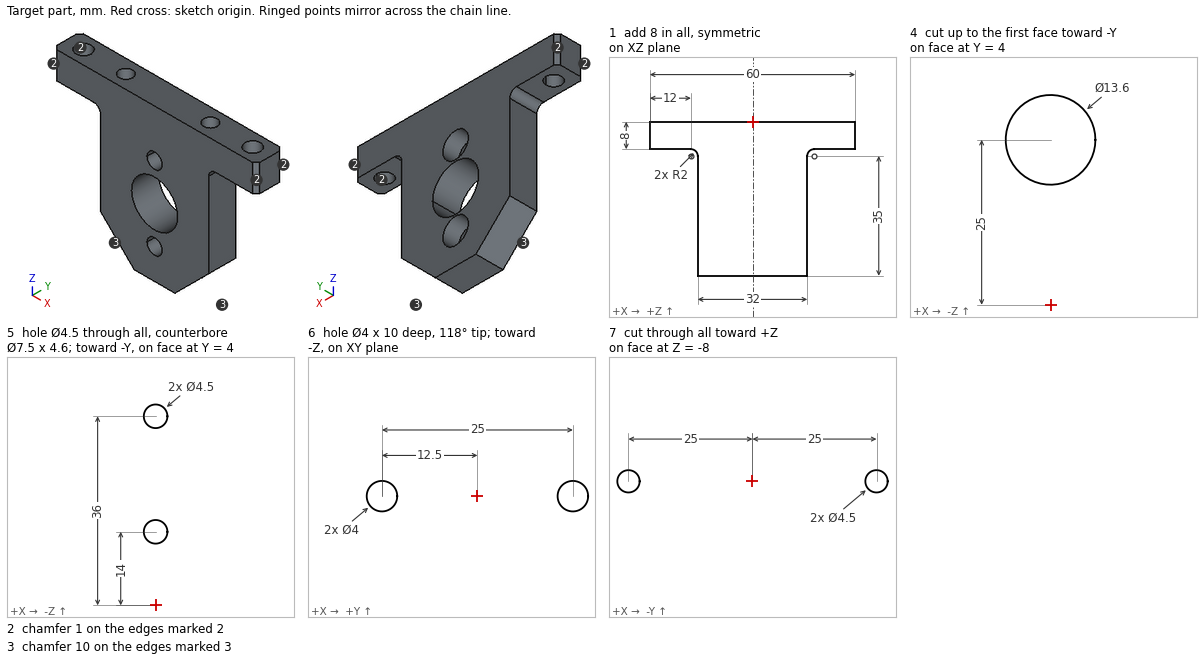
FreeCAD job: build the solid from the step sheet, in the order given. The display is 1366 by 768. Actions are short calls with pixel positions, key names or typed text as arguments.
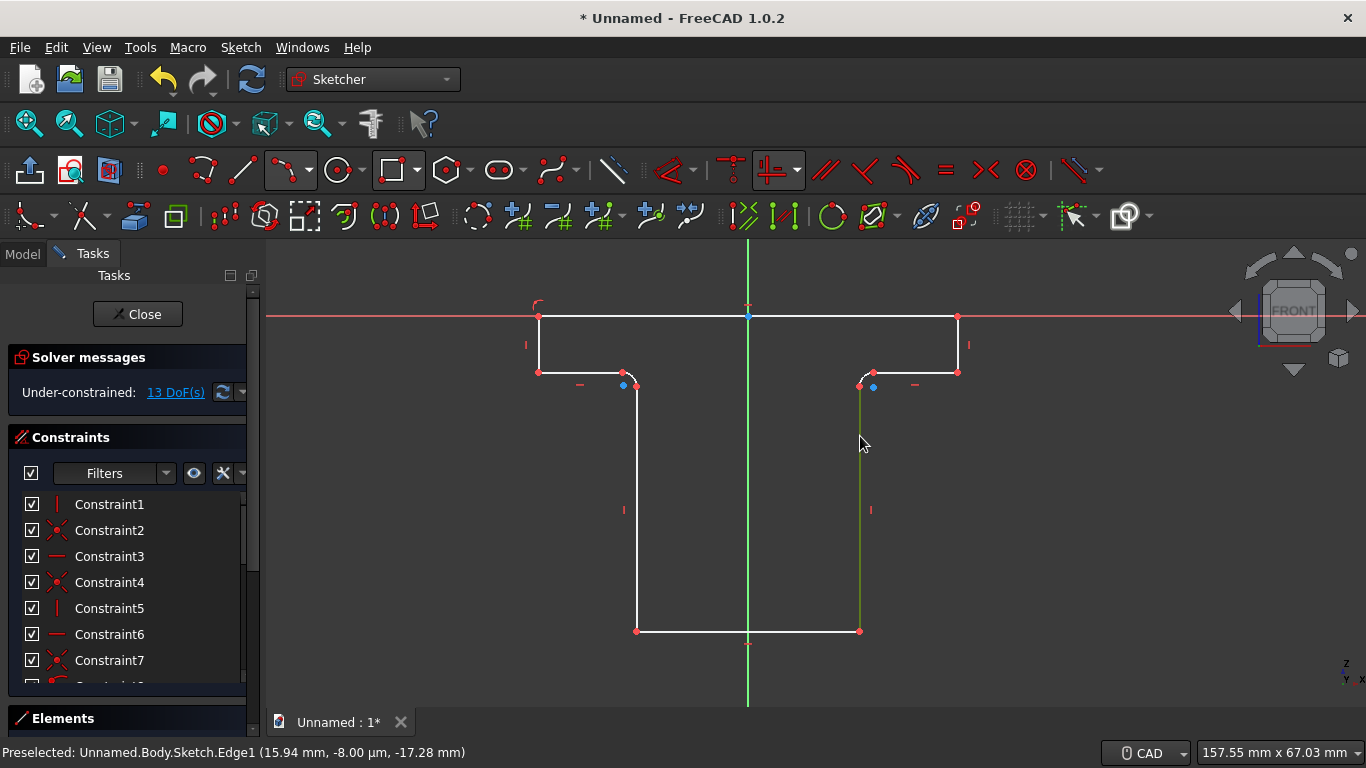
scroll(864, 377, up, 2)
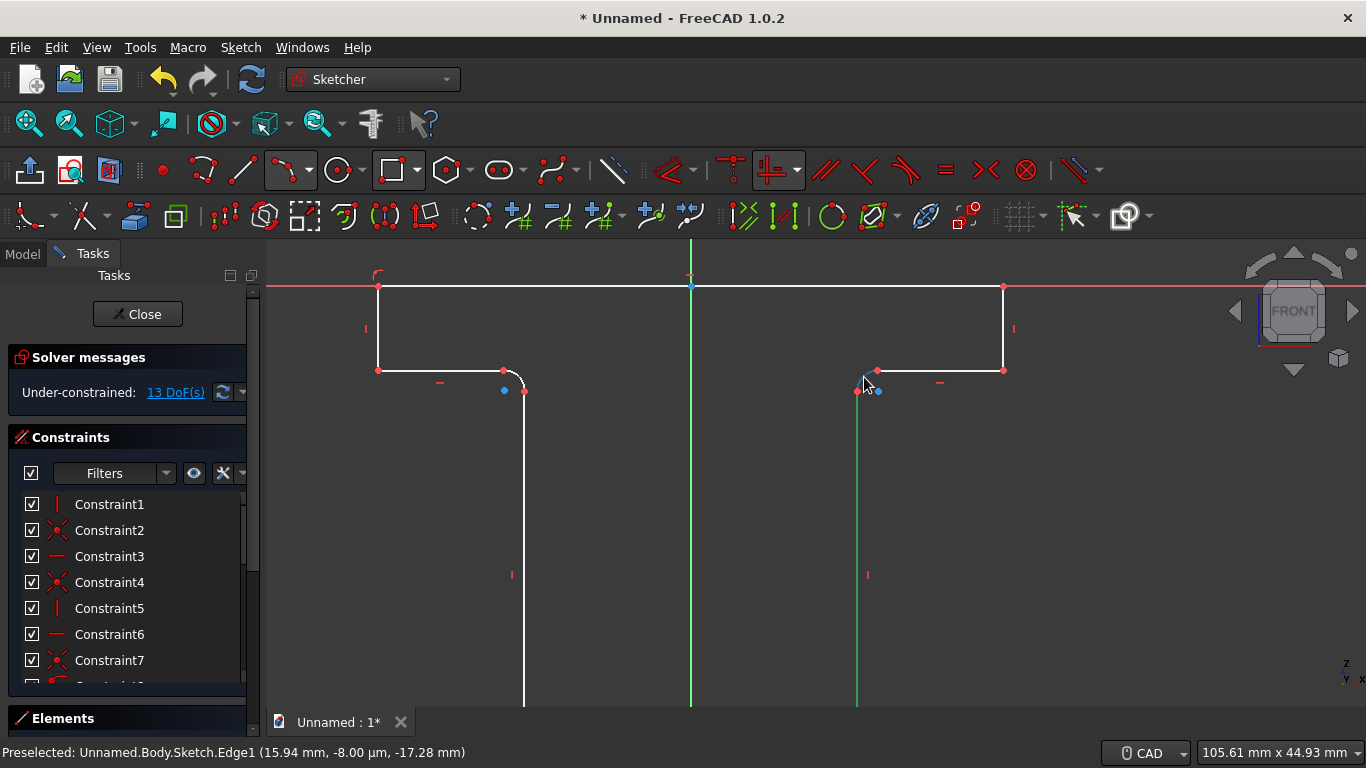
click(863, 377)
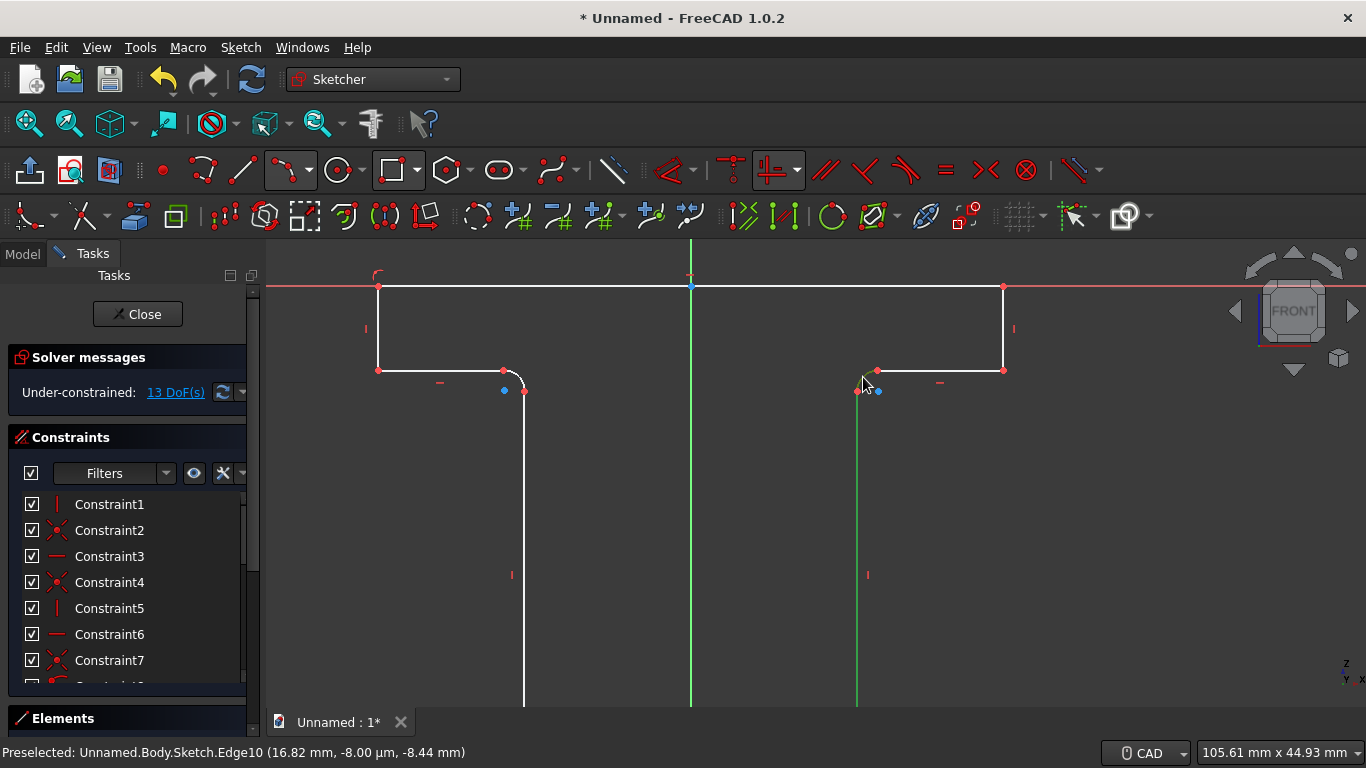
click(906, 170)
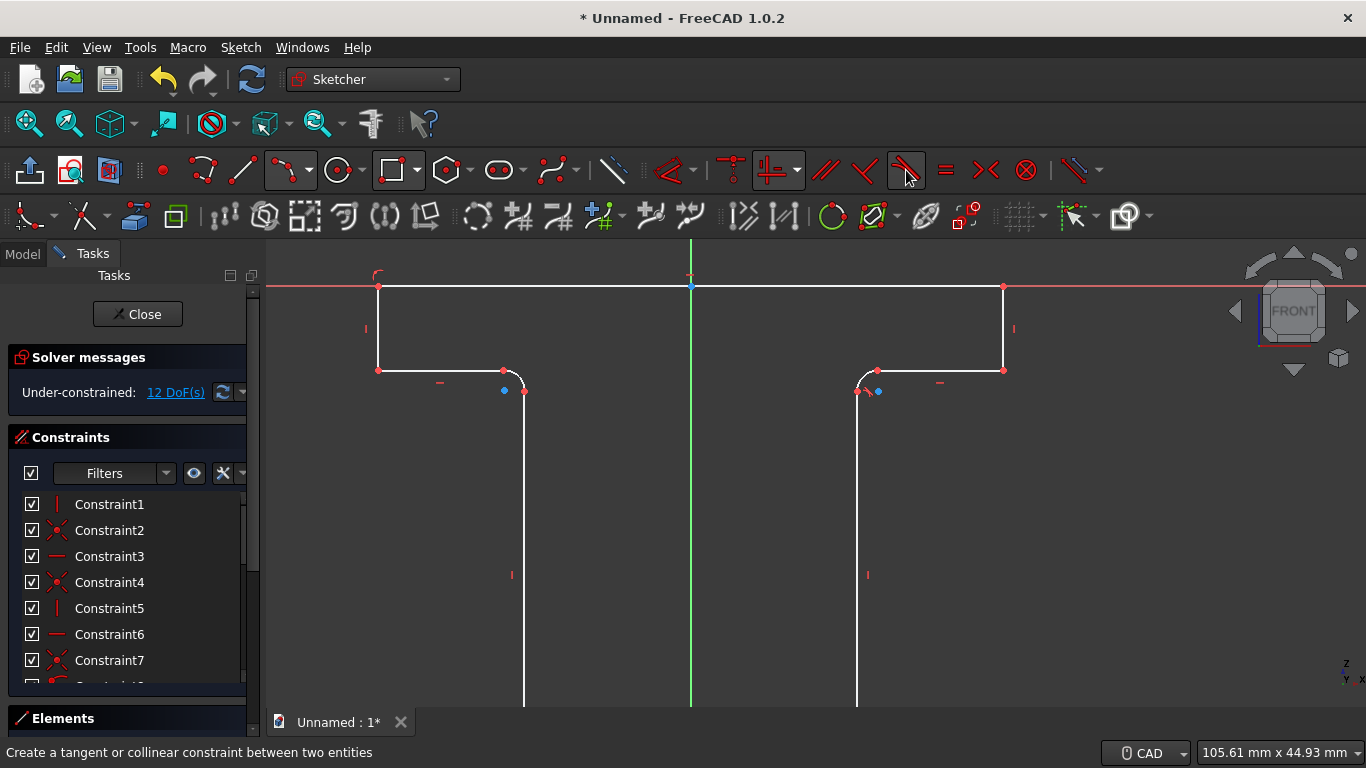
click(524, 647)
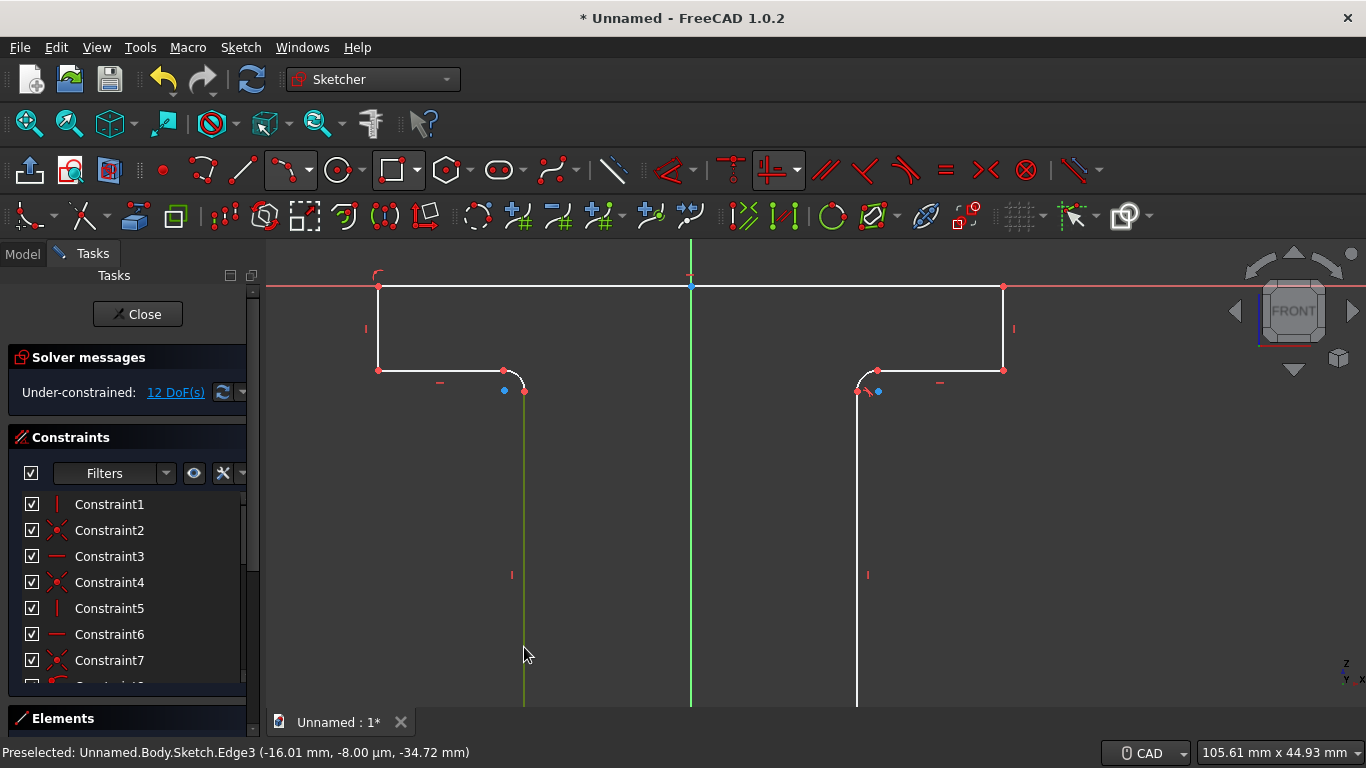
scroll(522, 382, up, 2)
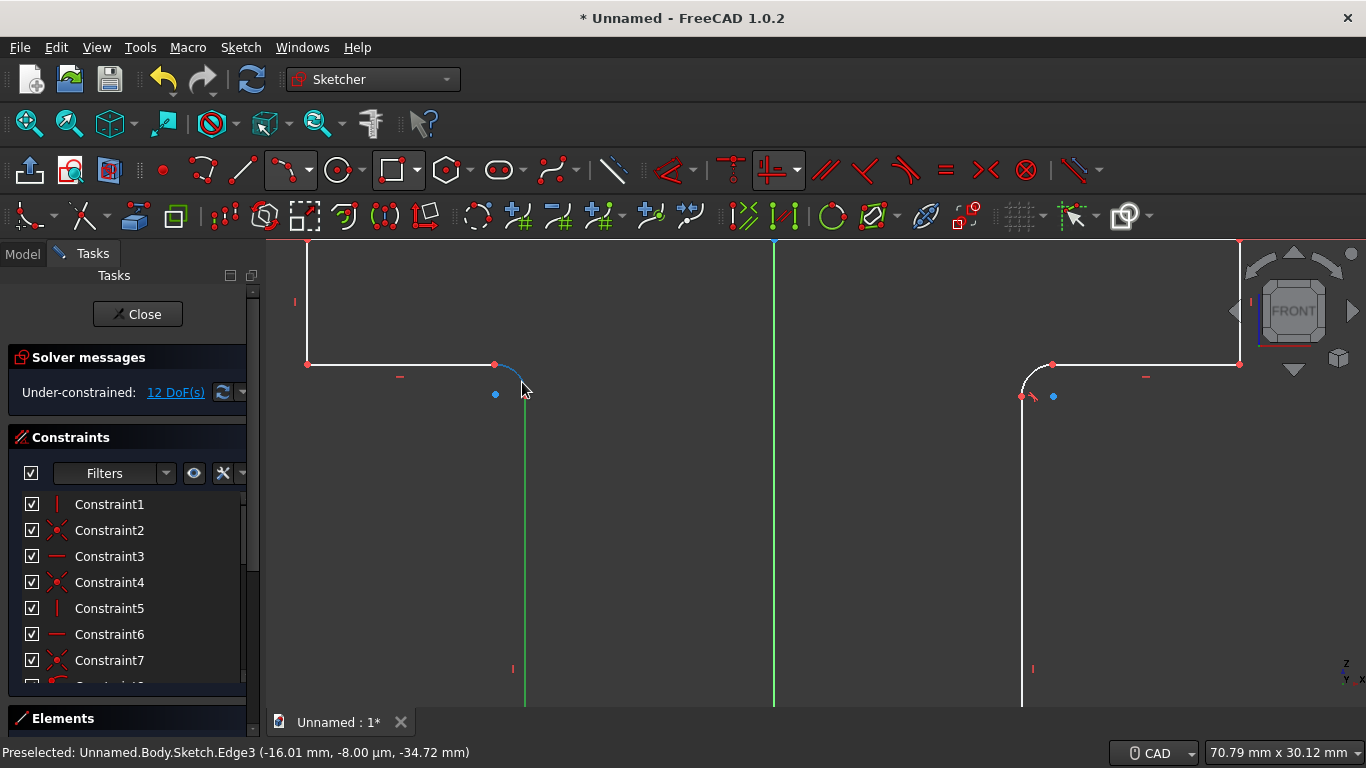
click(523, 381)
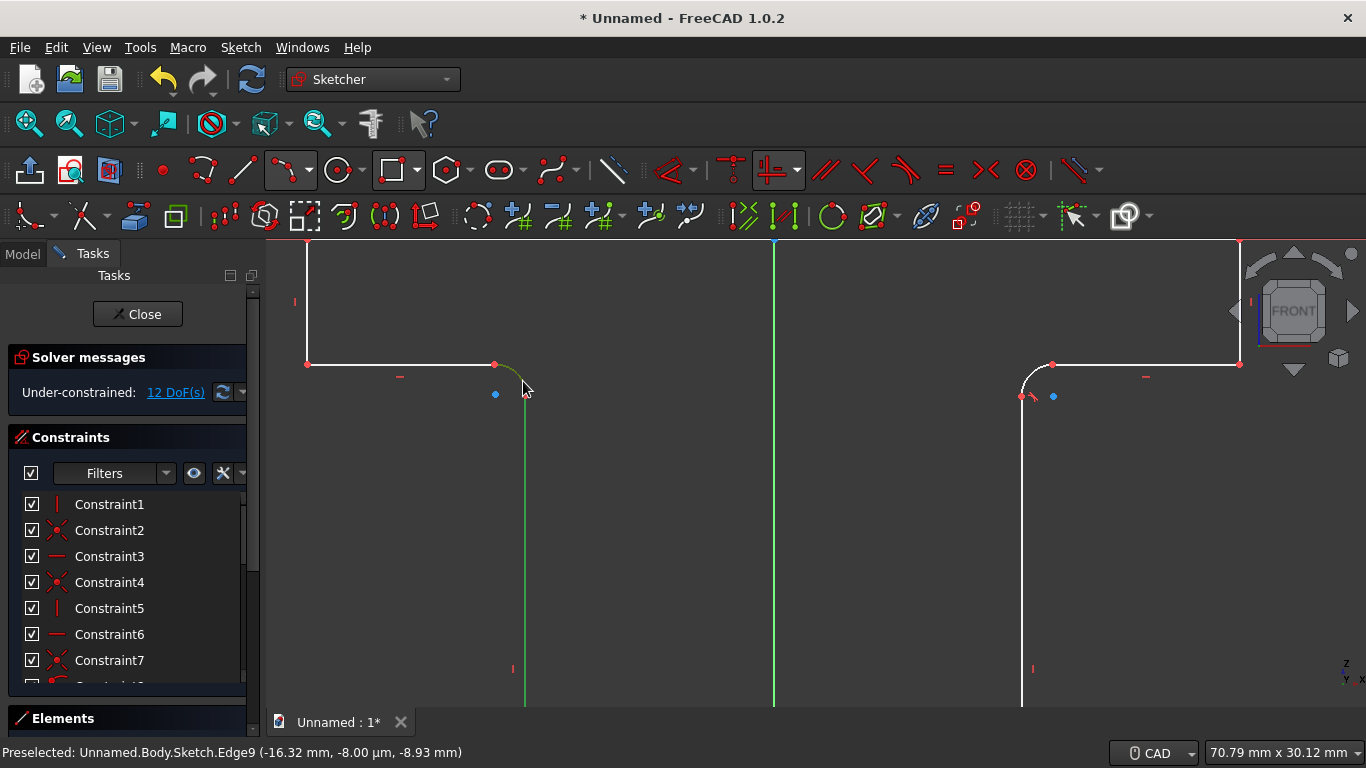
click(906, 170)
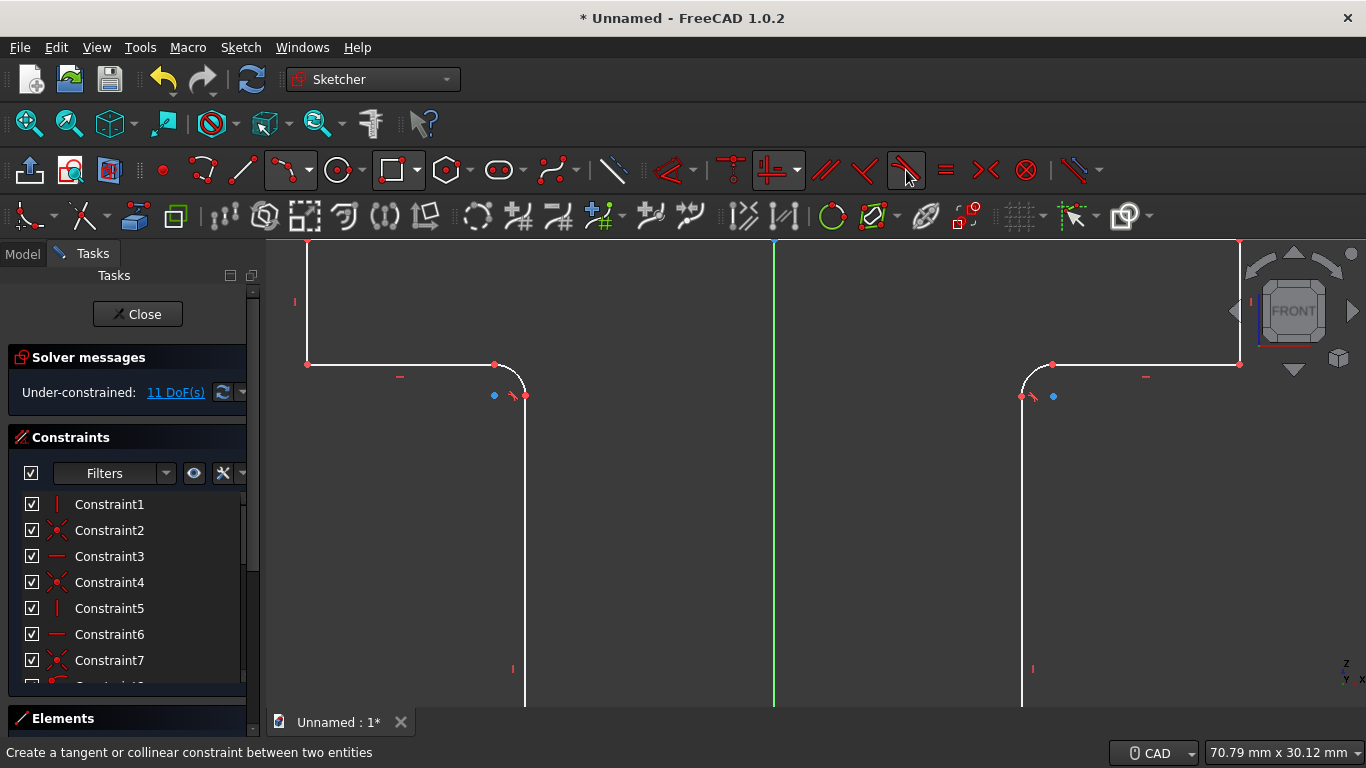
click(438, 365)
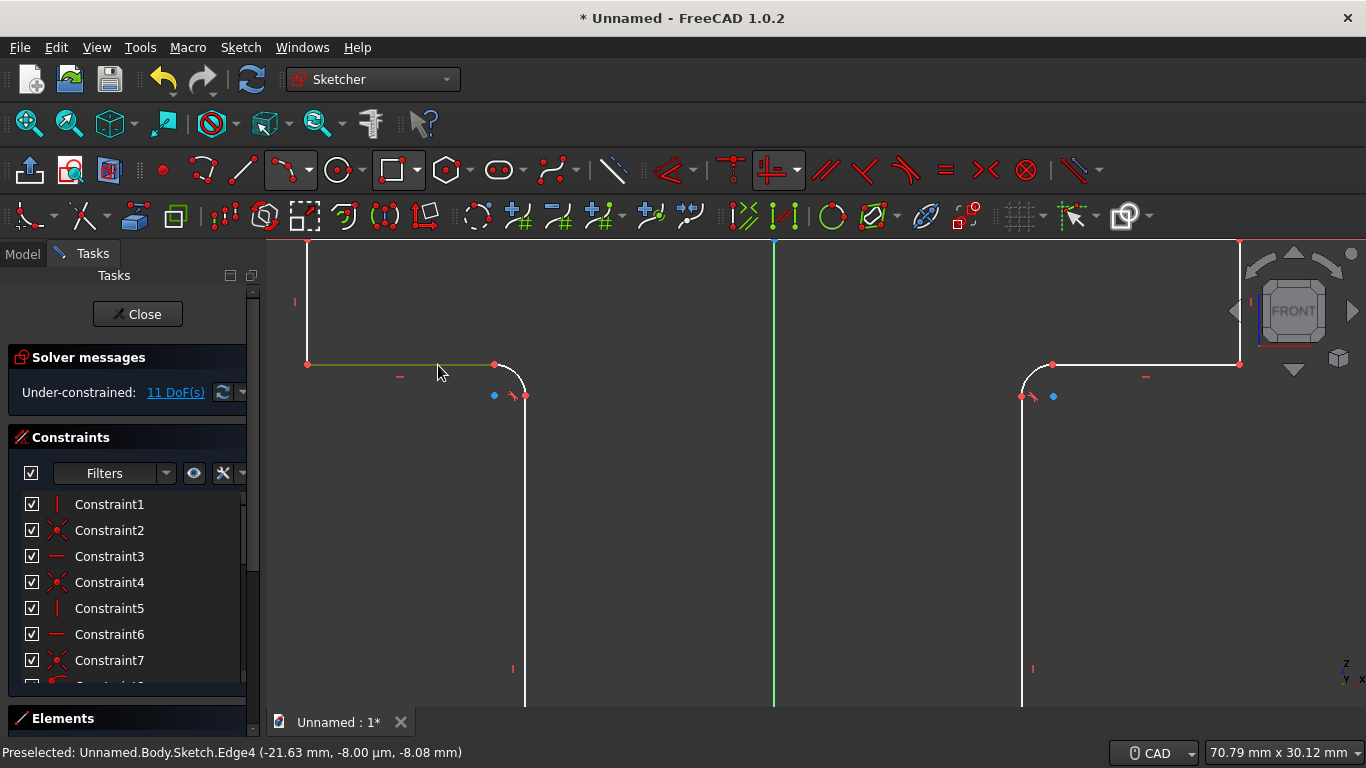
click(522, 382)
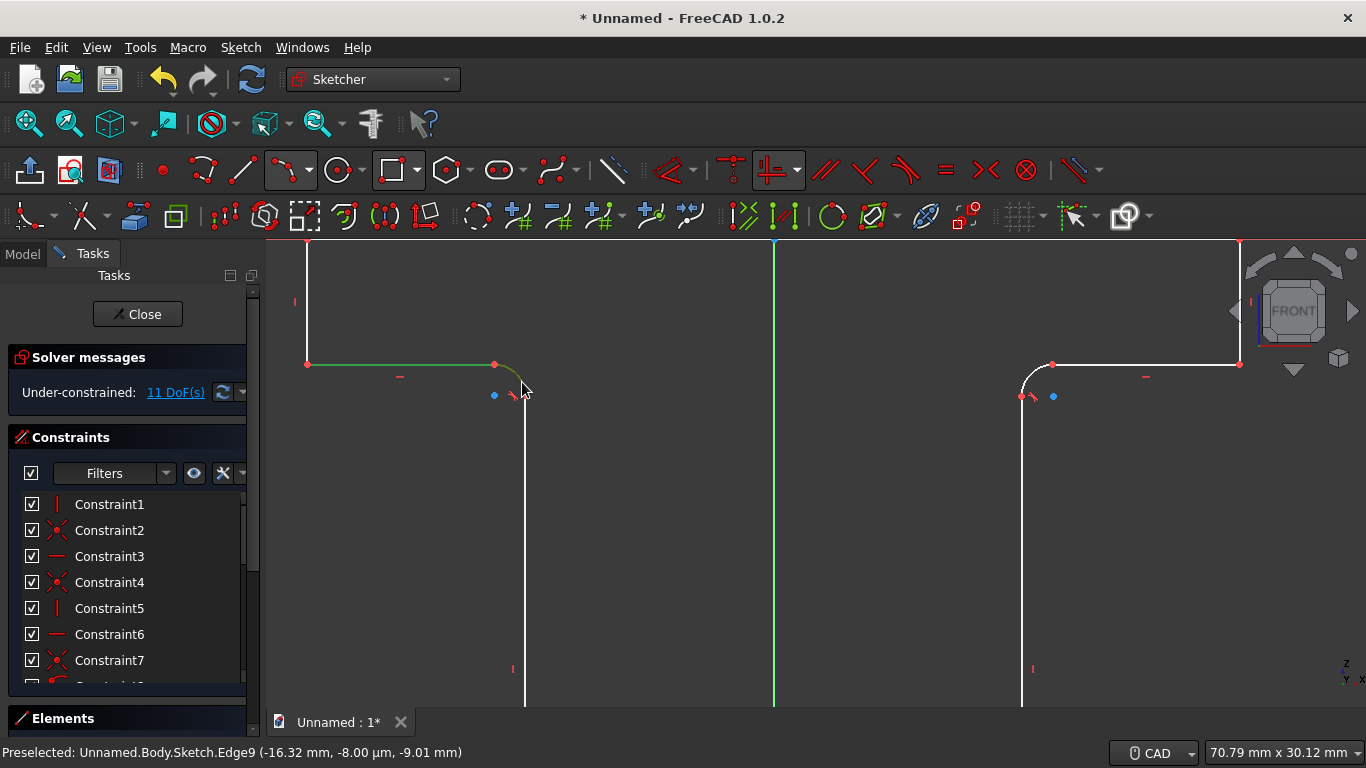
click(906, 170)